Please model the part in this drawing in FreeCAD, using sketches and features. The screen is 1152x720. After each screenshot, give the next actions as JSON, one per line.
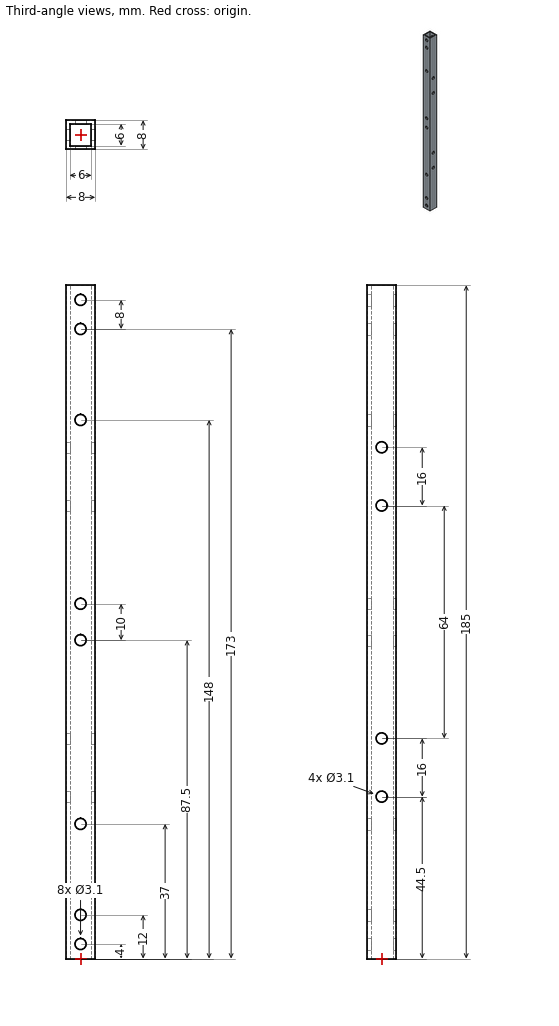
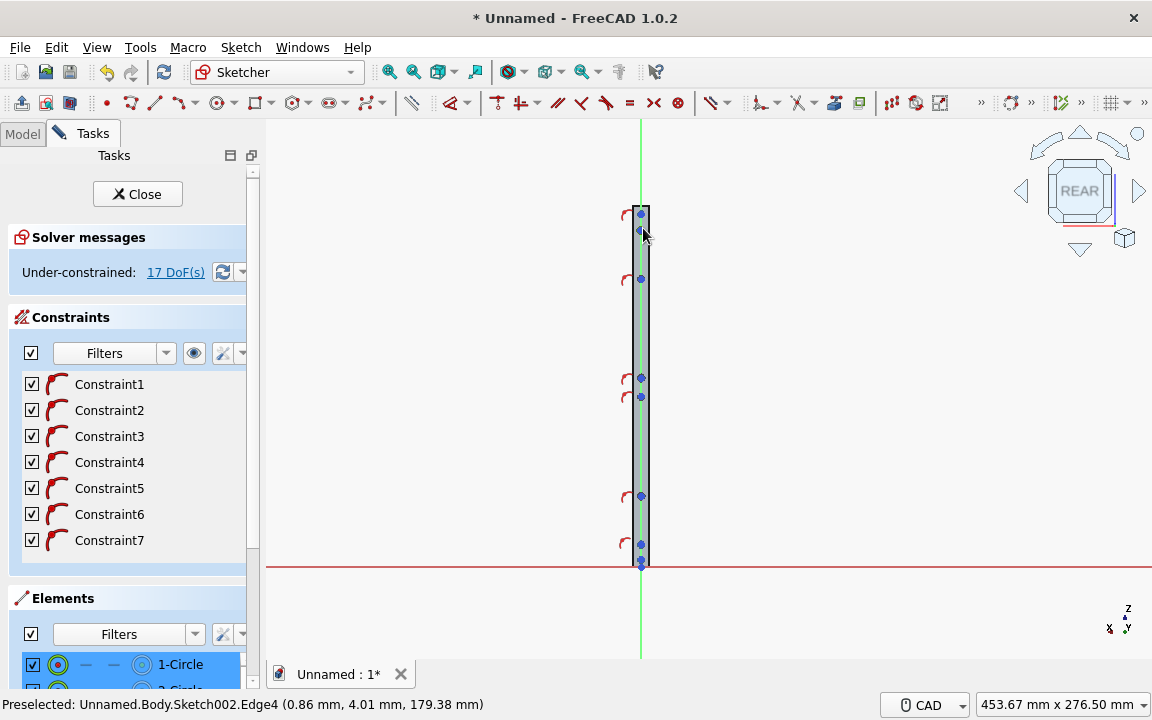
{"action": "scroll", "coordinate": [643, 395], "scroll_direction": "up", "scroll_amount": 10}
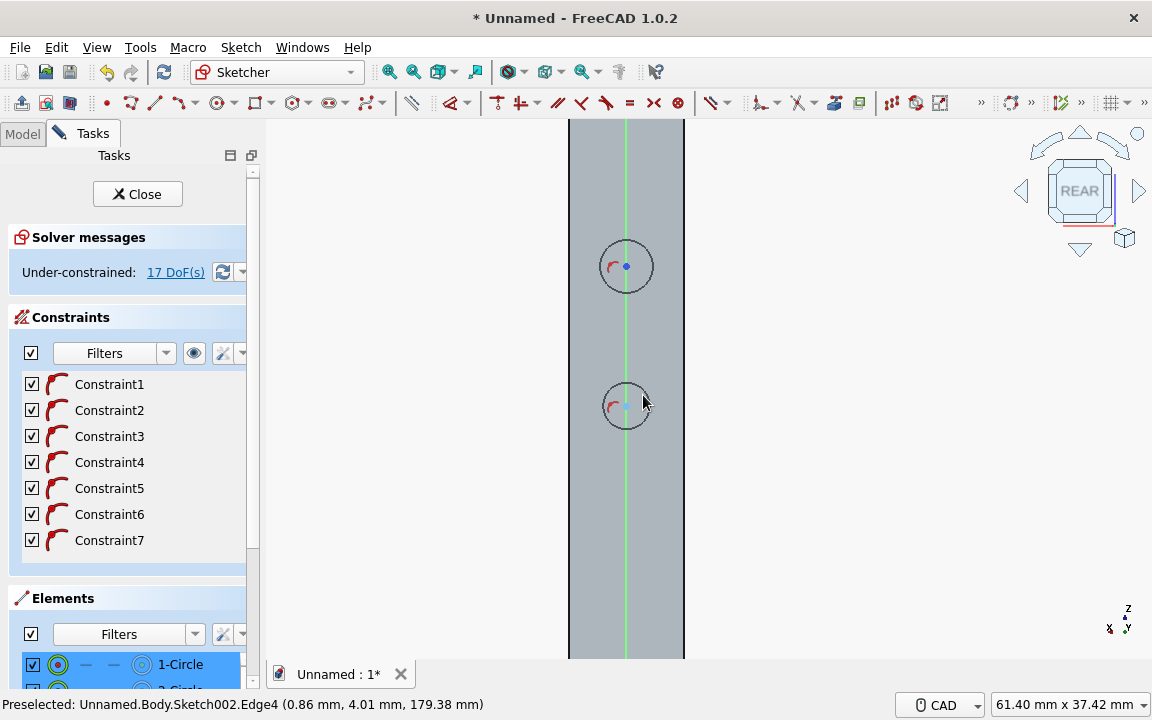
{"action": "left_click", "coordinate": [643, 390]}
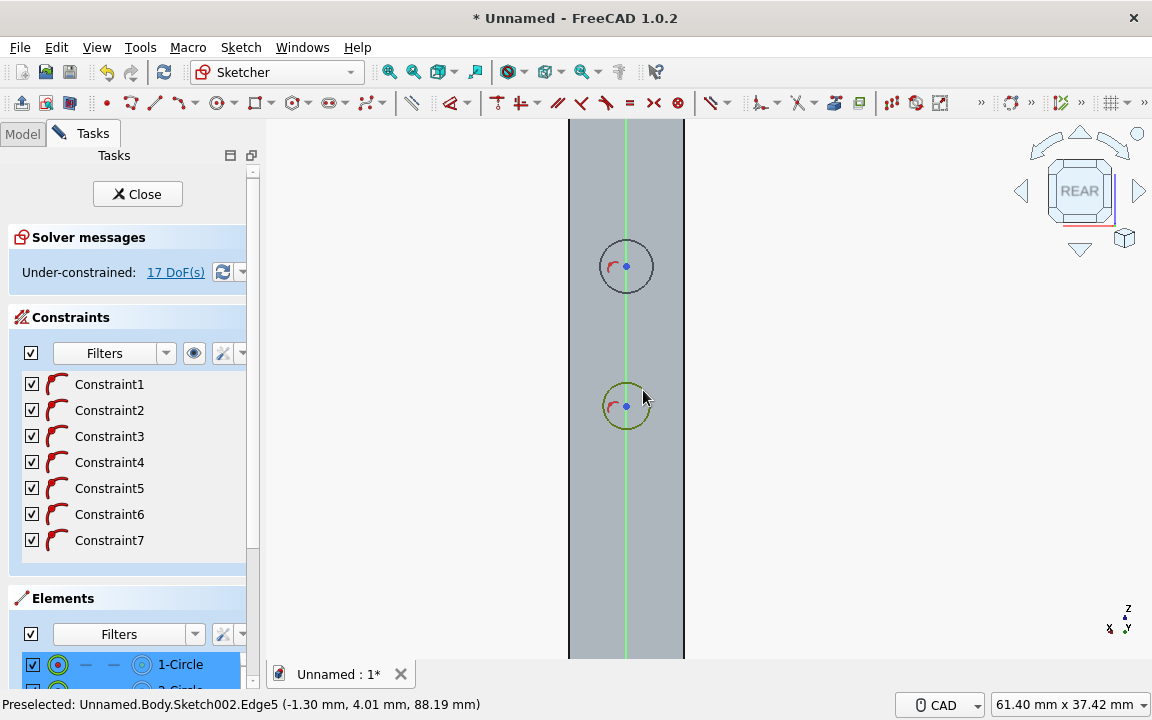
{"action": "left_click", "coordinate": [645, 248]}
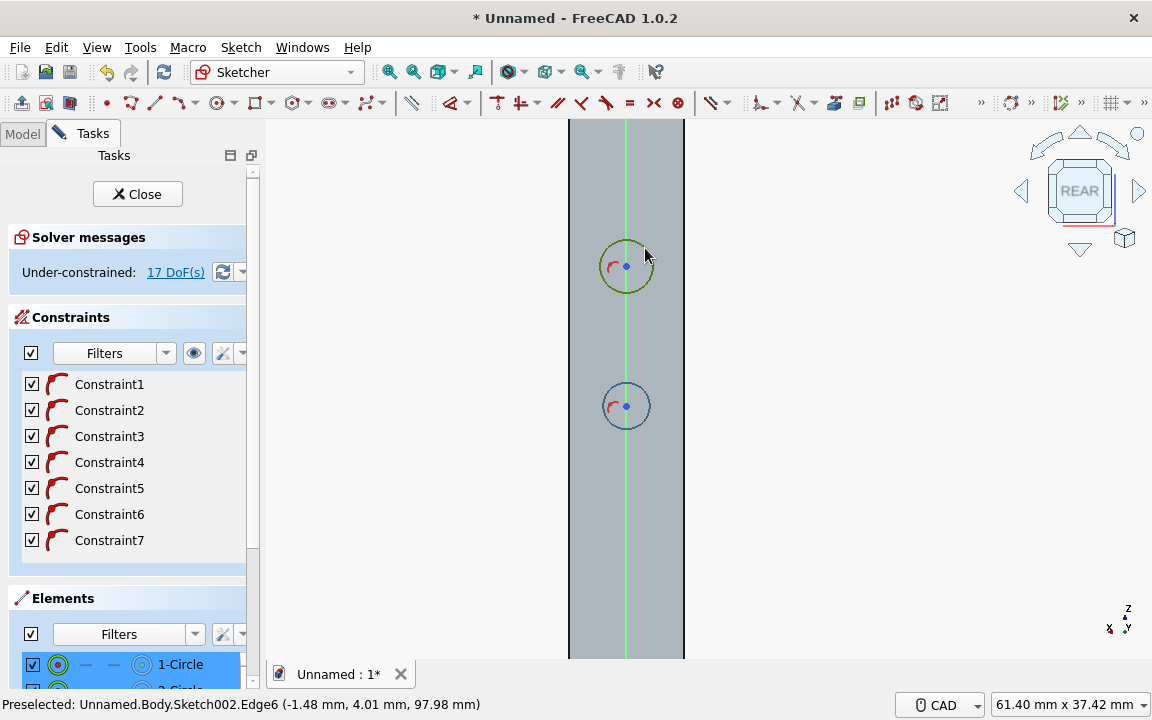
{"action": "scroll", "coordinate": [643, 395], "scroll_direction": "down", "scroll_amount": 10}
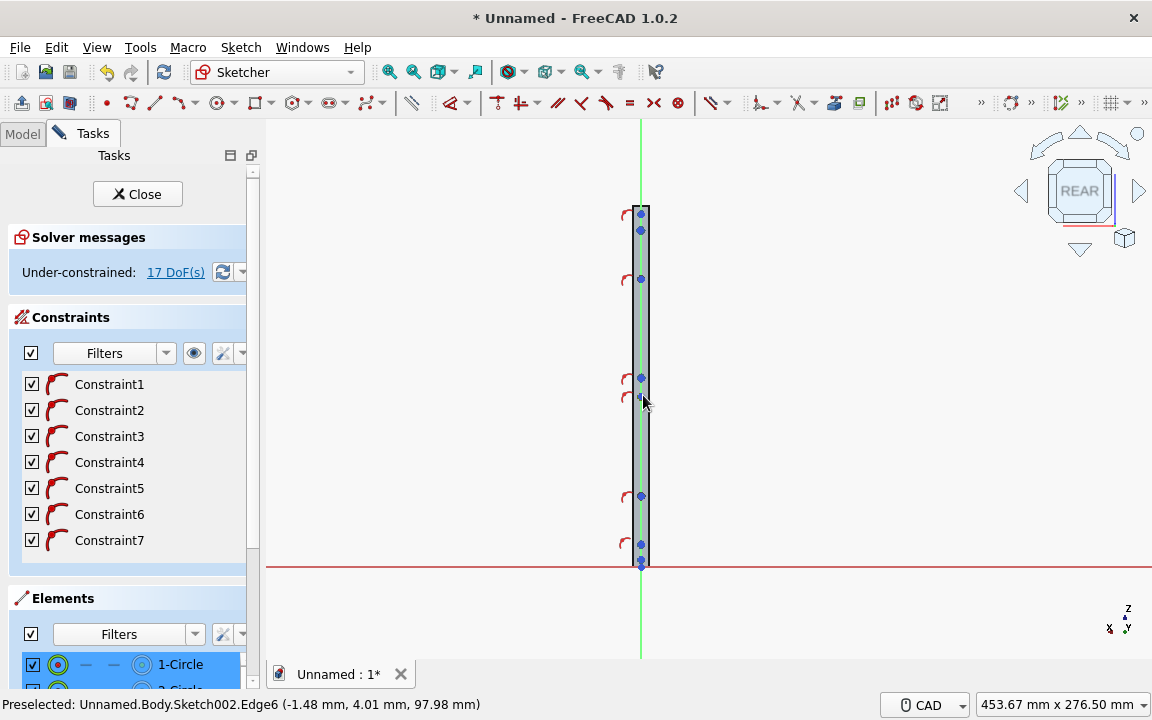
{"action": "scroll", "coordinate": [643, 277], "scroll_direction": "up", "scroll_amount": 9}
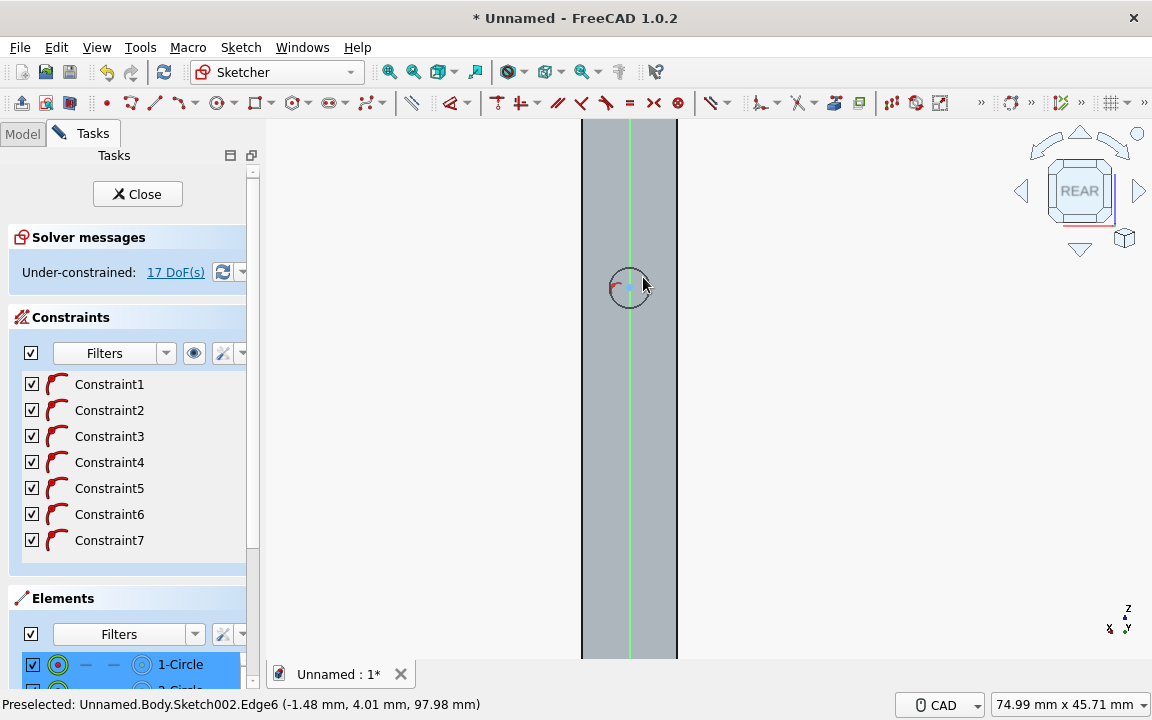
{"action": "left_click", "coordinate": [644, 274]}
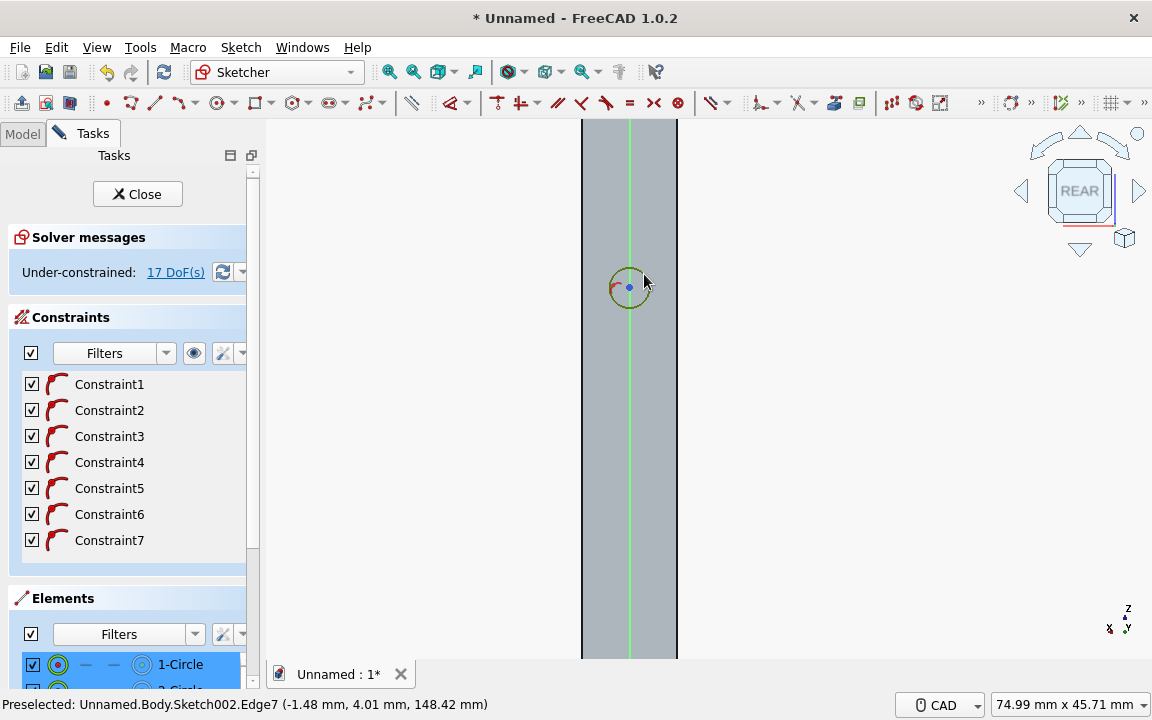
{"action": "scroll", "coordinate": [643, 277], "scroll_direction": "down", "scroll_amount": 9}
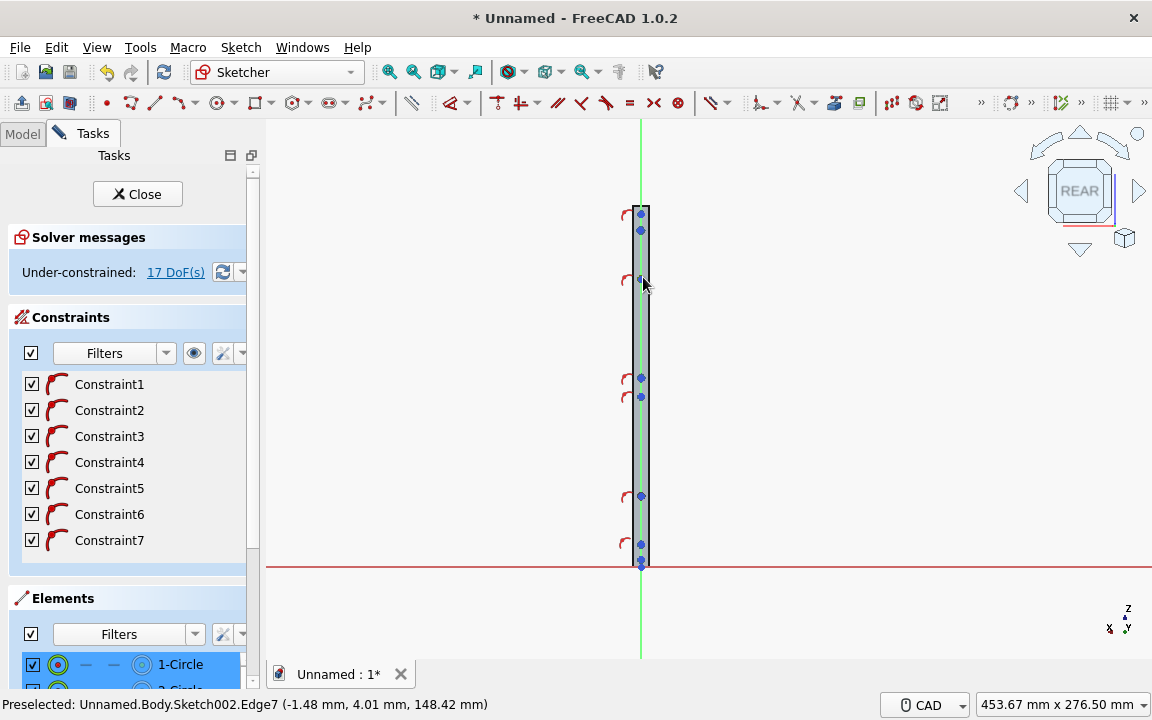
{"action": "scroll", "coordinate": [644, 494], "scroll_direction": "up", "scroll_amount": 9}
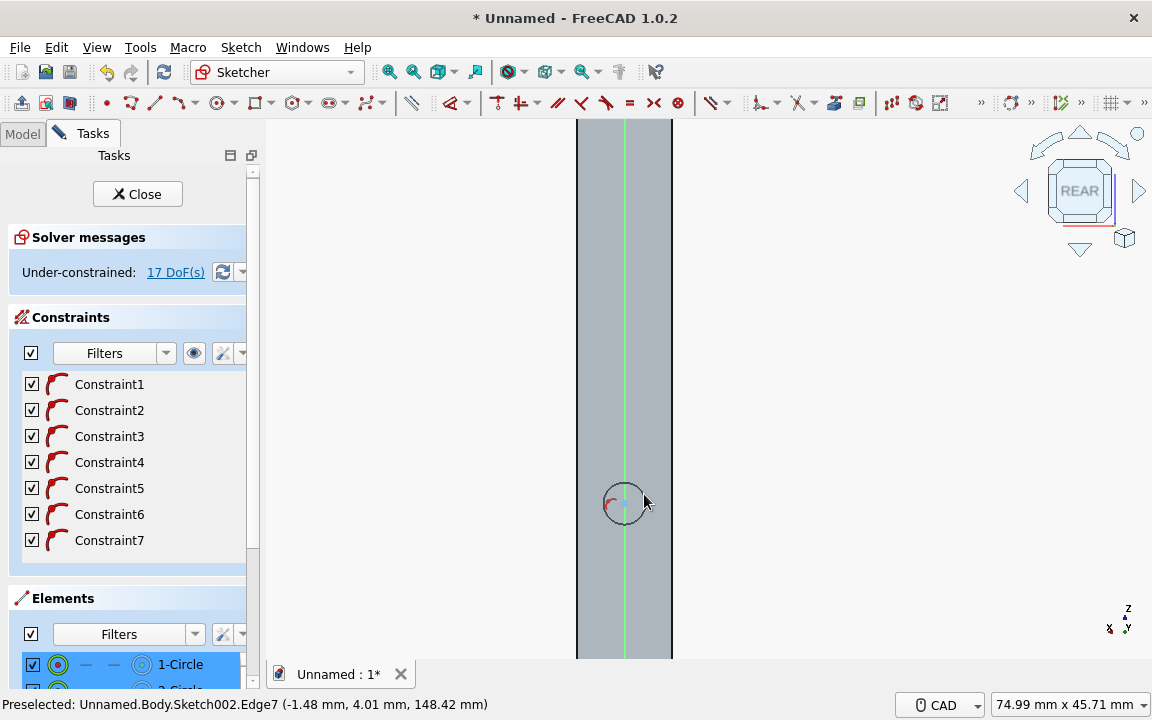
{"action": "left_click", "coordinate": [639, 489]}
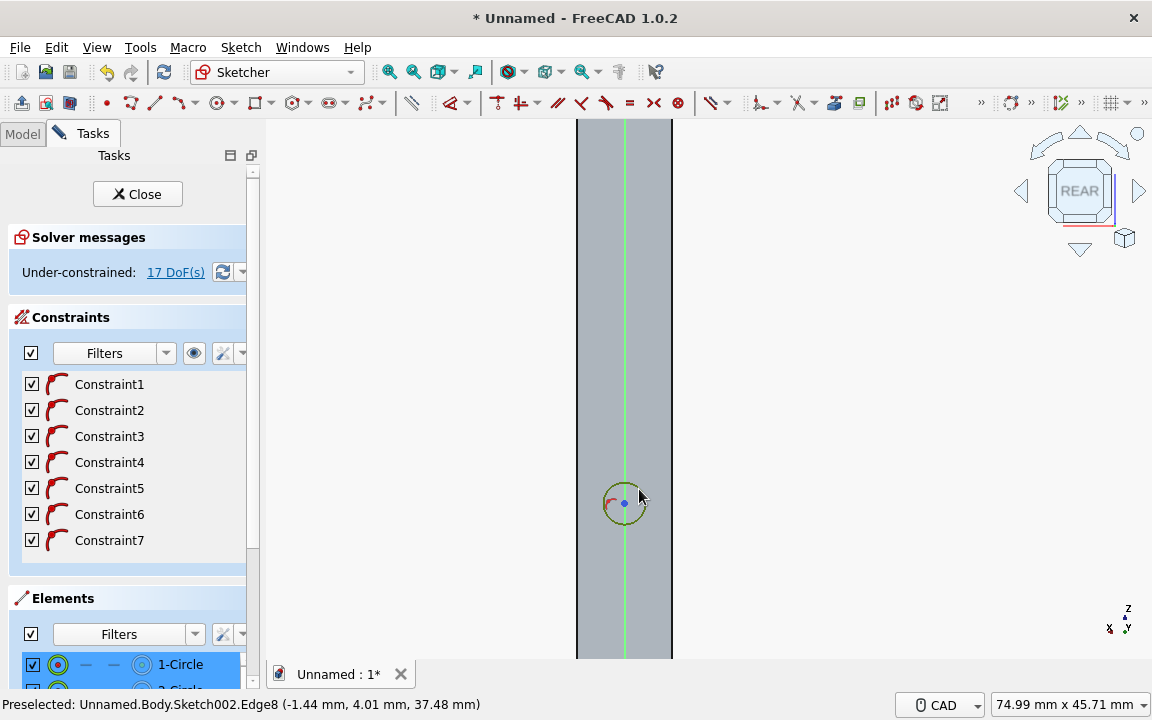
{"action": "left_click", "coordinate": [630, 104]}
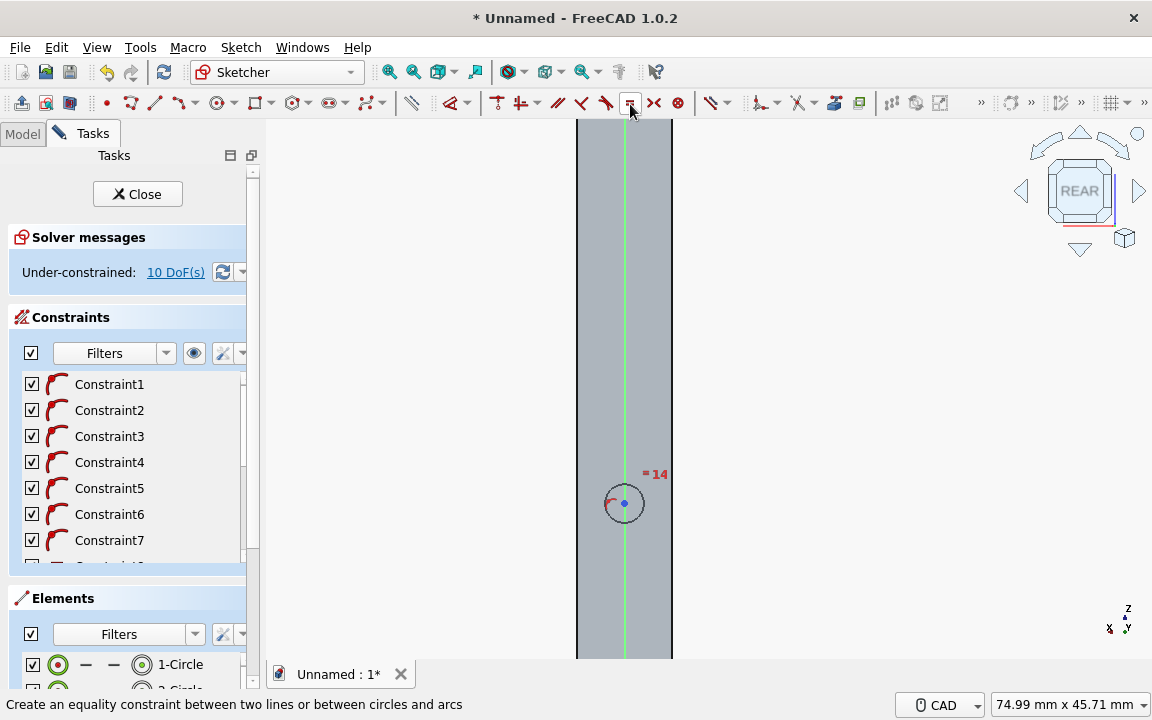
{"action": "scroll", "coordinate": [644, 495], "scroll_direction": "down", "scroll_amount": 9}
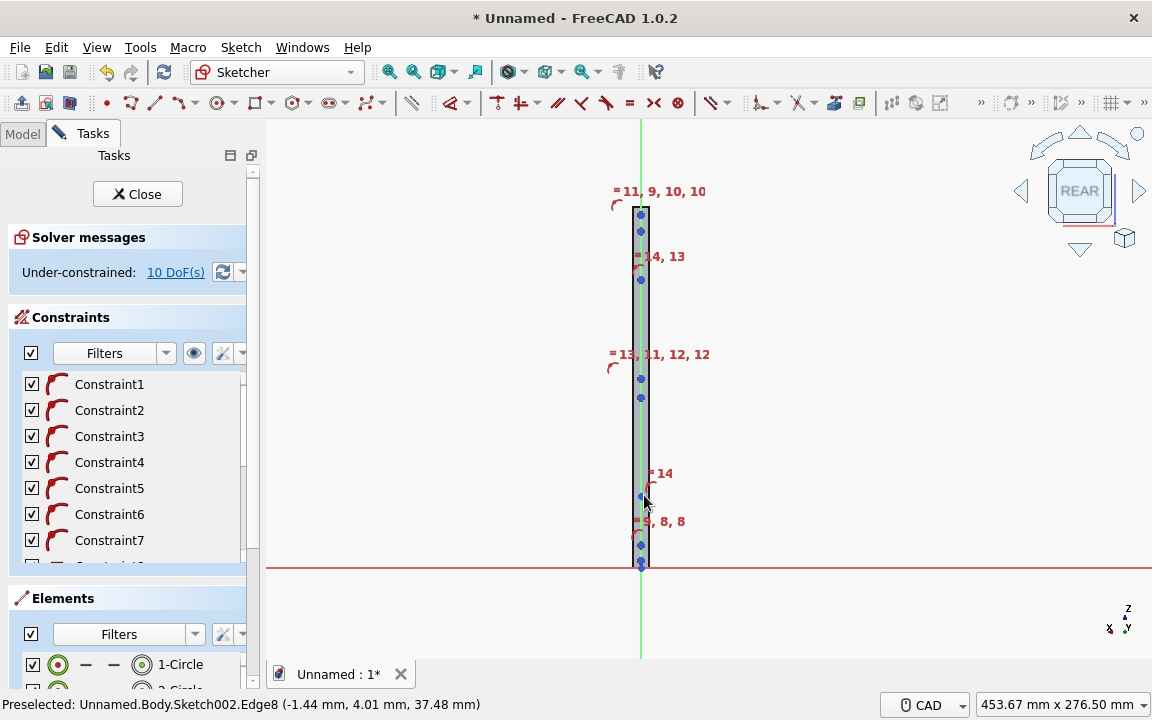
{"action": "left_click", "coordinate": [641, 231]}